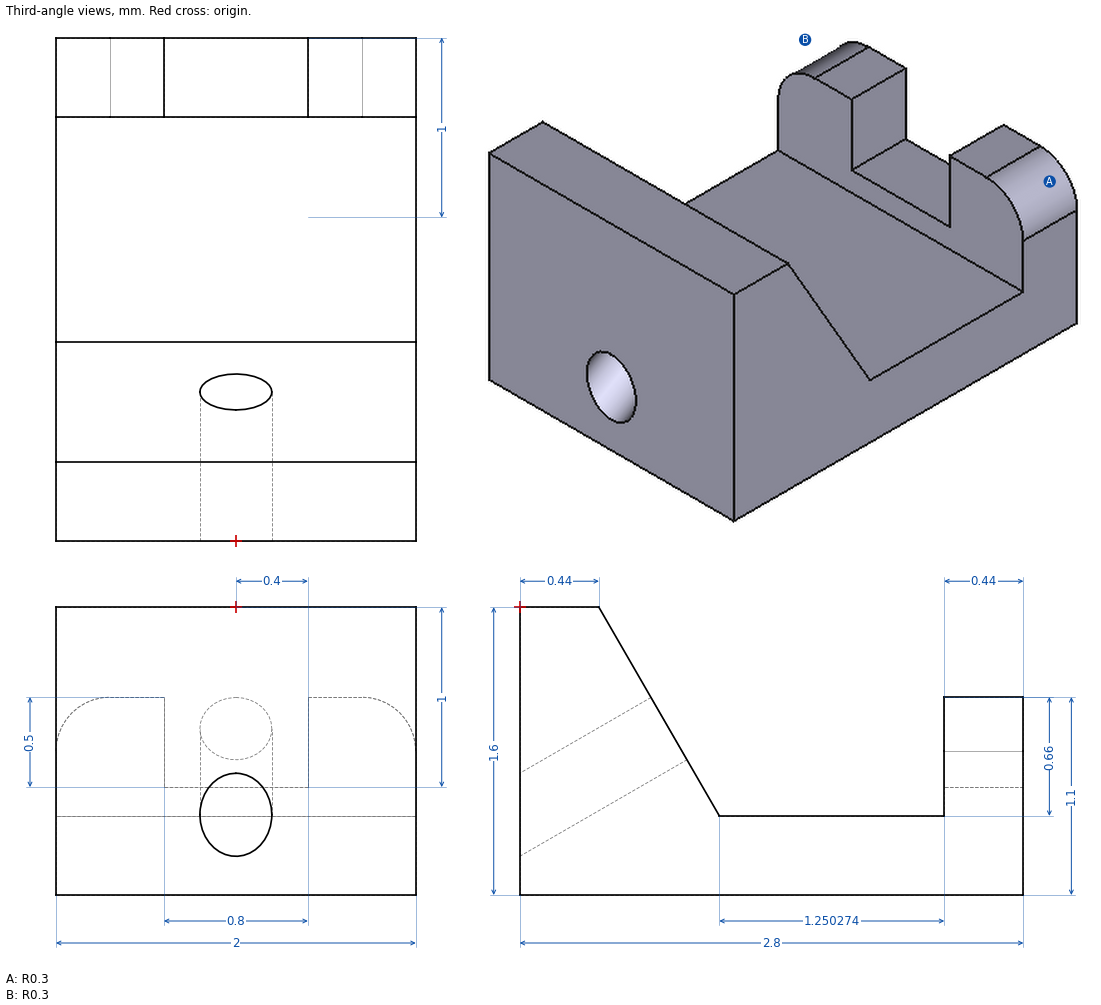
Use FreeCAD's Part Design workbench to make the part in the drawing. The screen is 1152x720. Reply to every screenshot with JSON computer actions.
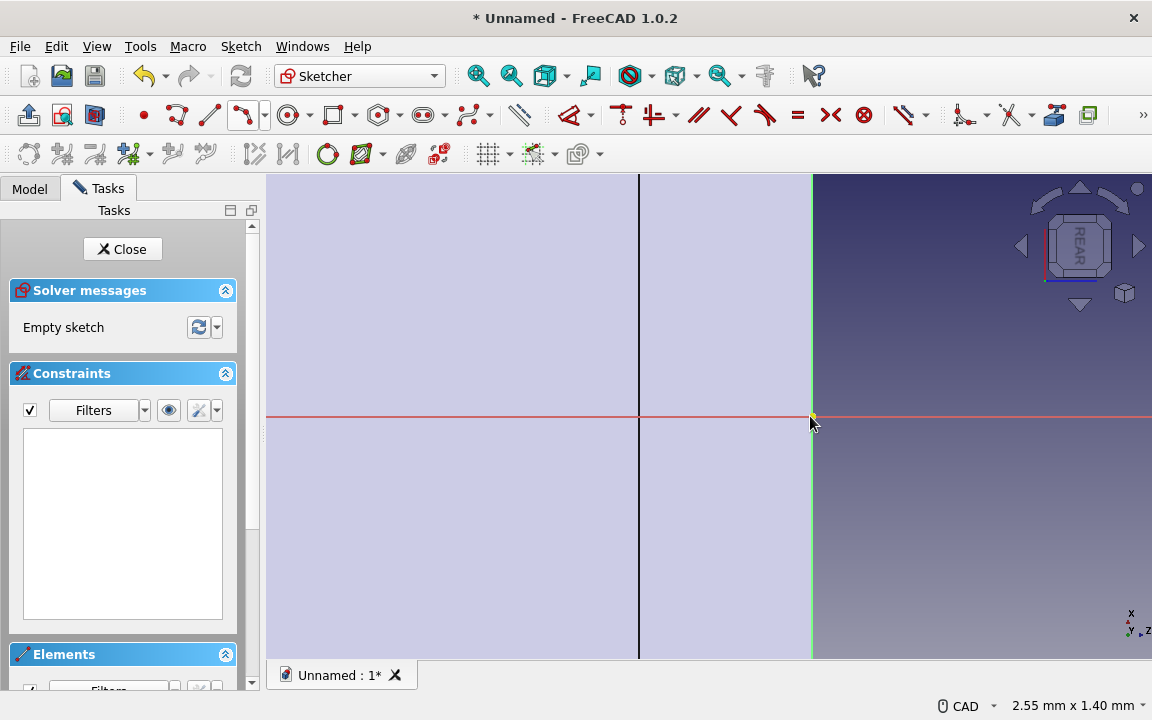
{"action": "left_click", "coordinate": [332, 116]}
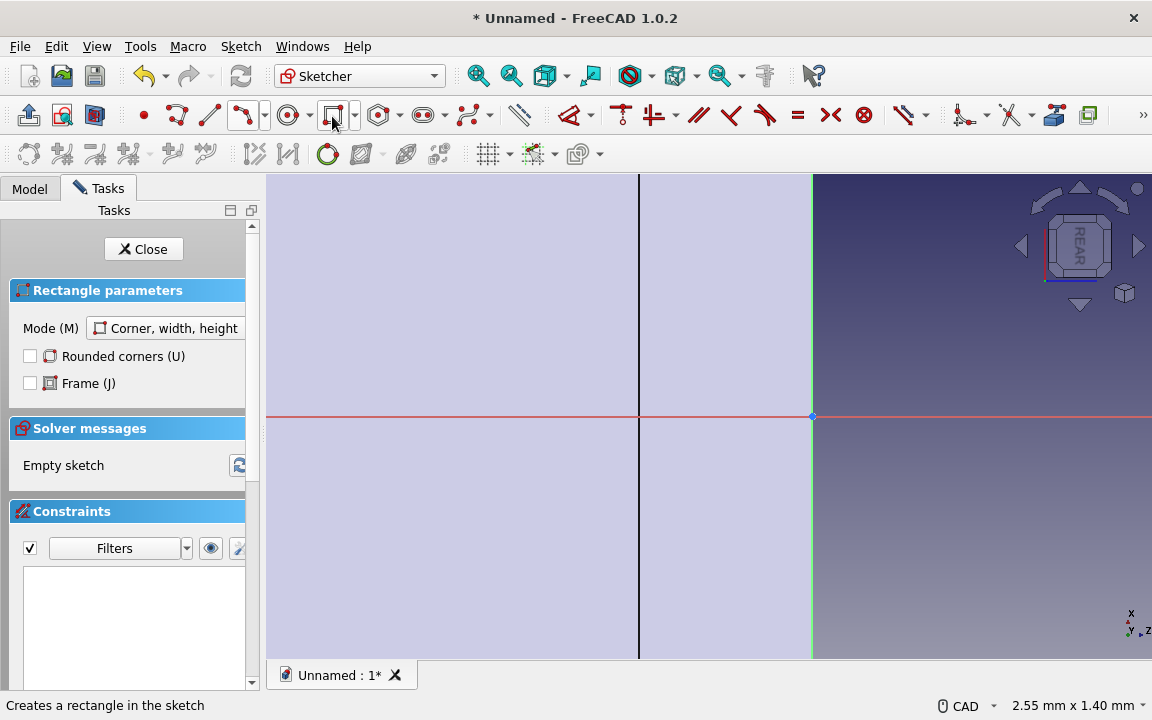
{"action": "left_click", "coordinate": [465, 278]}
{"action": "left_click", "coordinate": [639, 555]}
{"action": "key", "text": "Escape"}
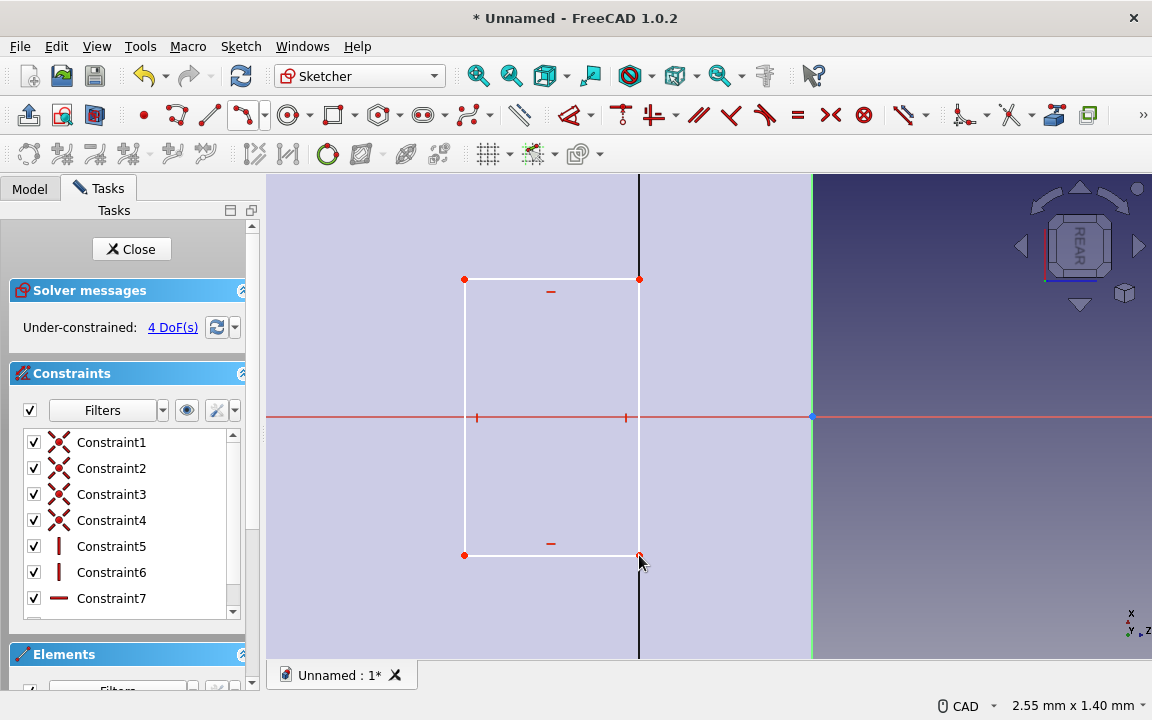
{"action": "left_click", "coordinate": [568, 116]}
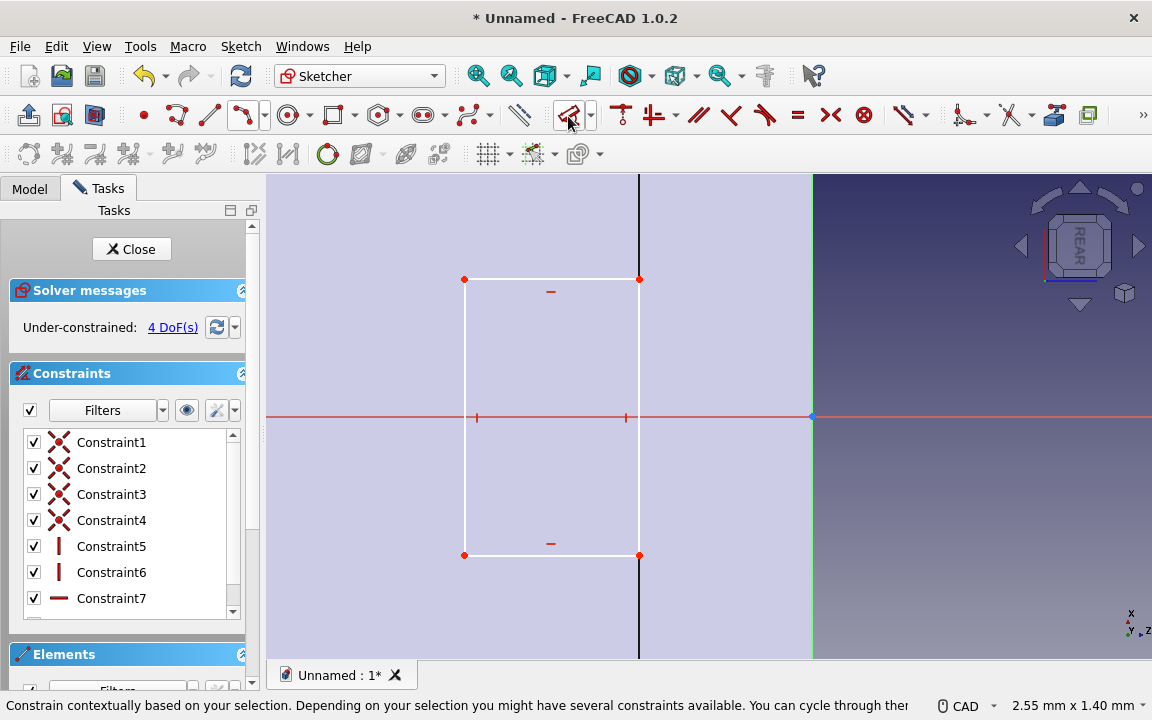
{"action": "left_click", "coordinate": [465, 279]}
{"action": "left_click", "coordinate": [639, 245]}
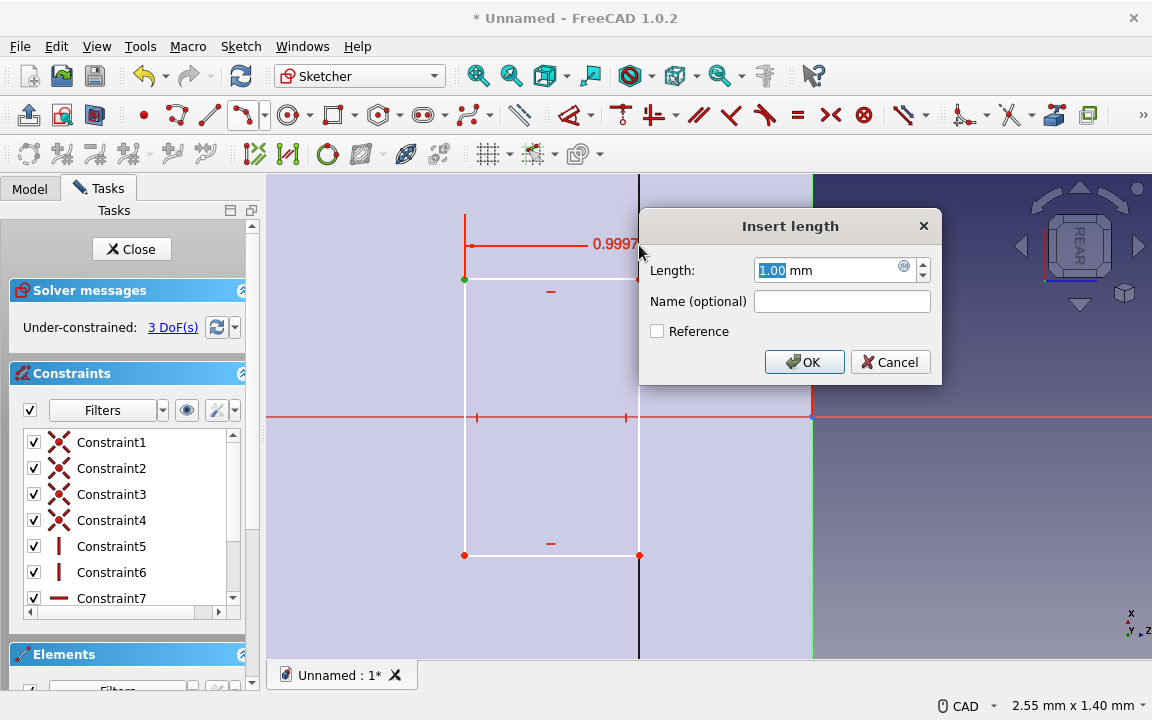
{"action": "type", "text": "1"}
{"action": "key", "text": "Return"}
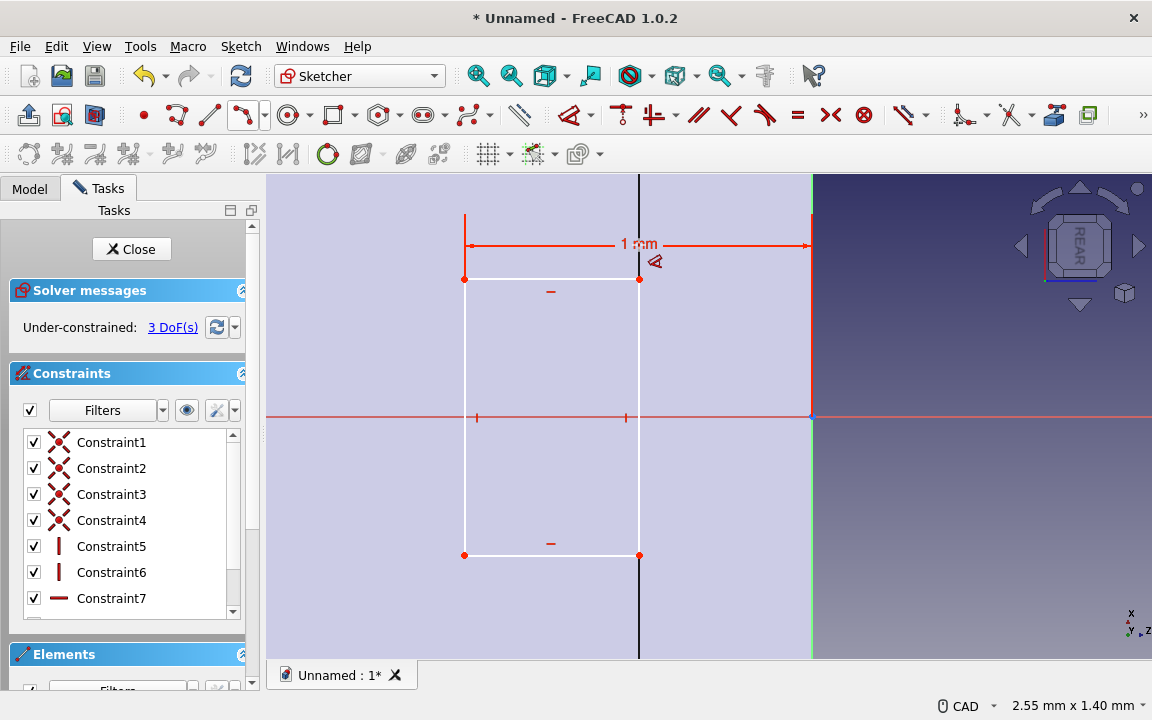
{"action": "left_click", "coordinate": [465, 362]}
{"action": "left_click", "coordinate": [431, 354]}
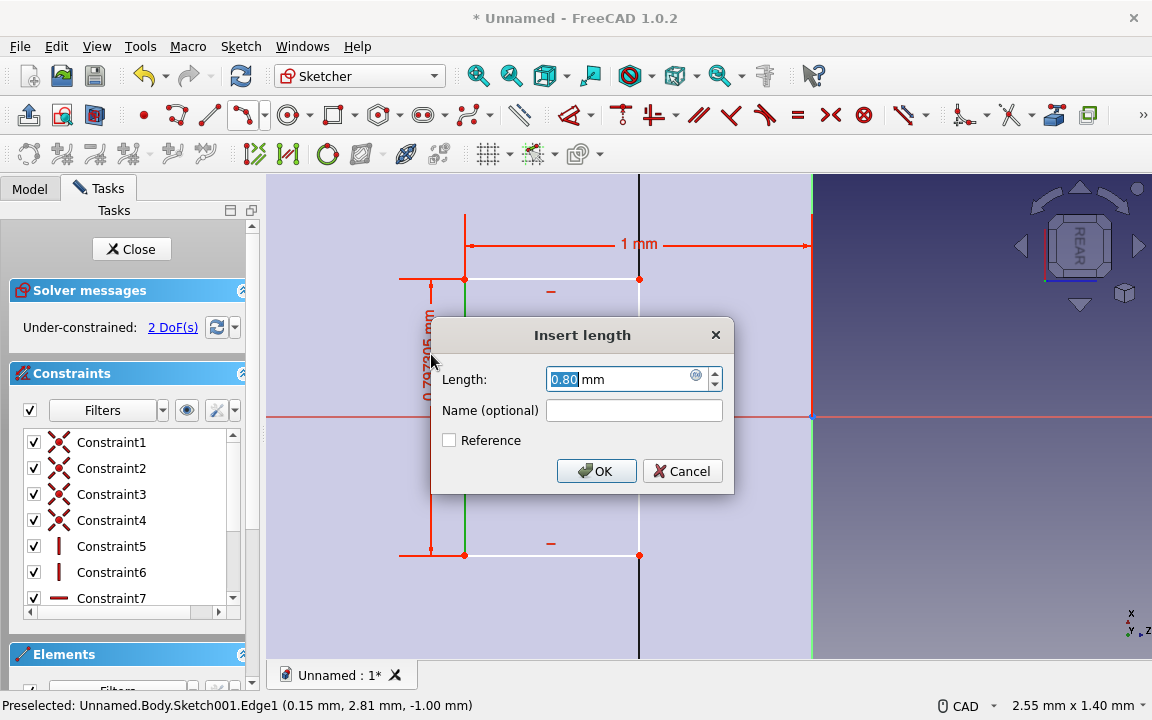
{"action": "type", "text": "0.8"}
{"action": "key", "text": "Return"}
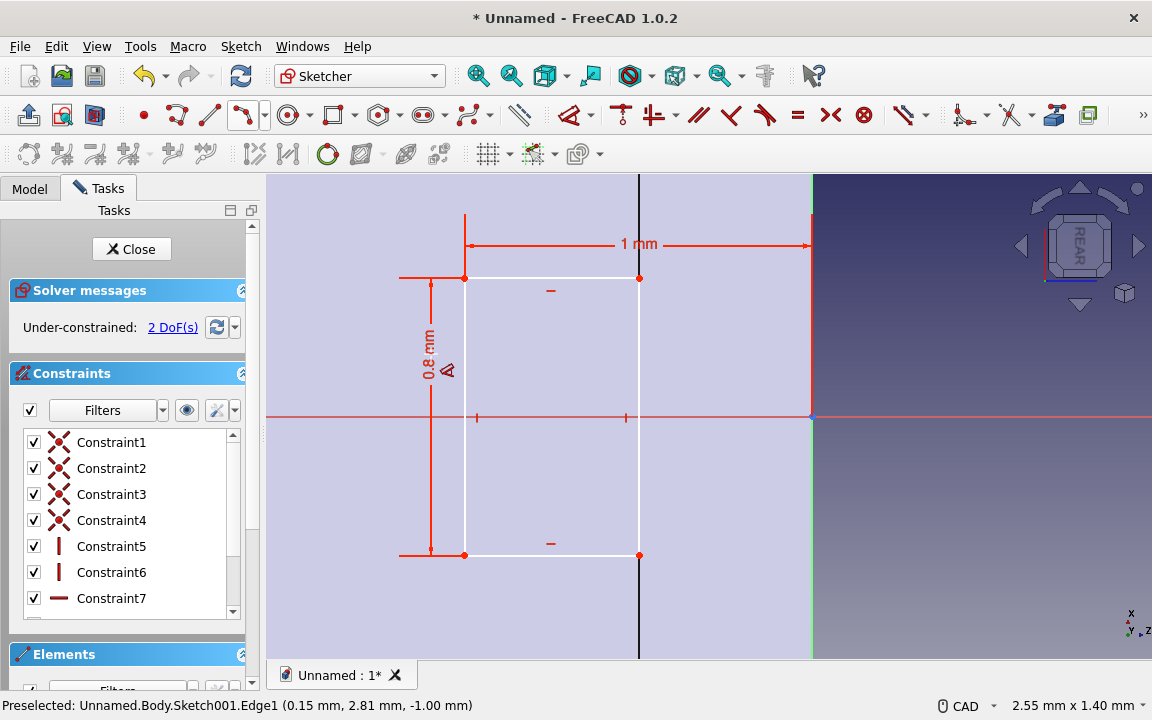
{"action": "left_click", "coordinate": [517, 556]}
{"action": "left_click", "coordinate": [552, 590]}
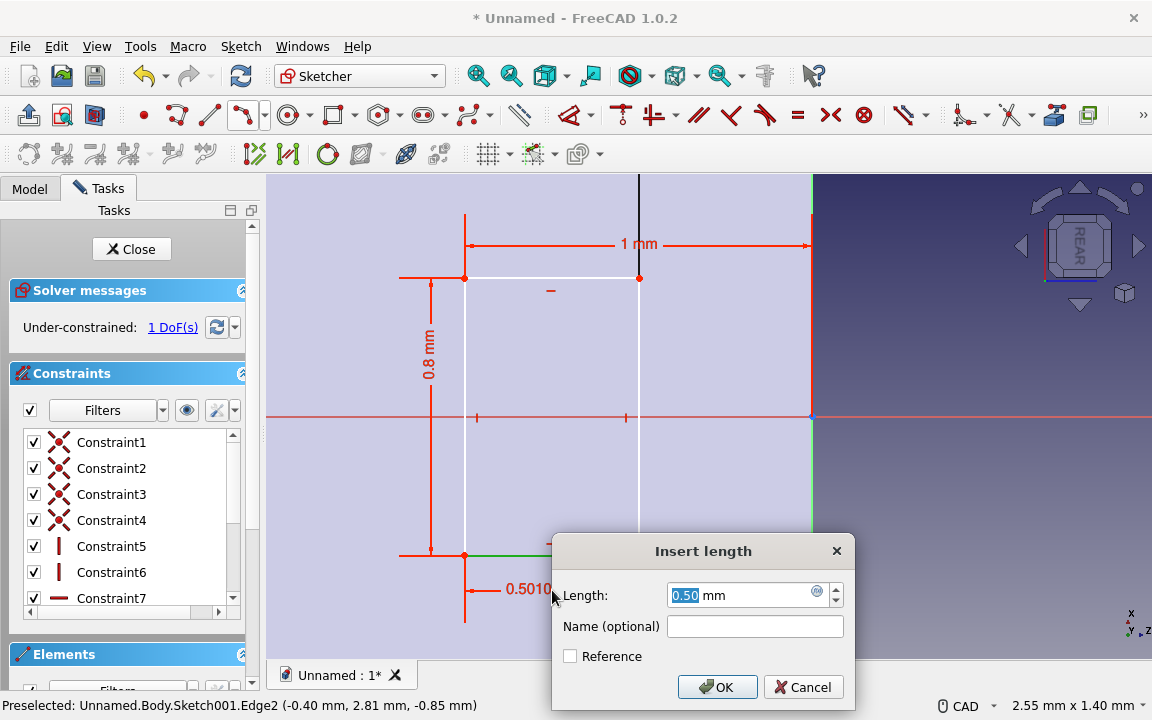
{"action": "type", "text": "0.5"}
{"action": "key", "text": "Return"}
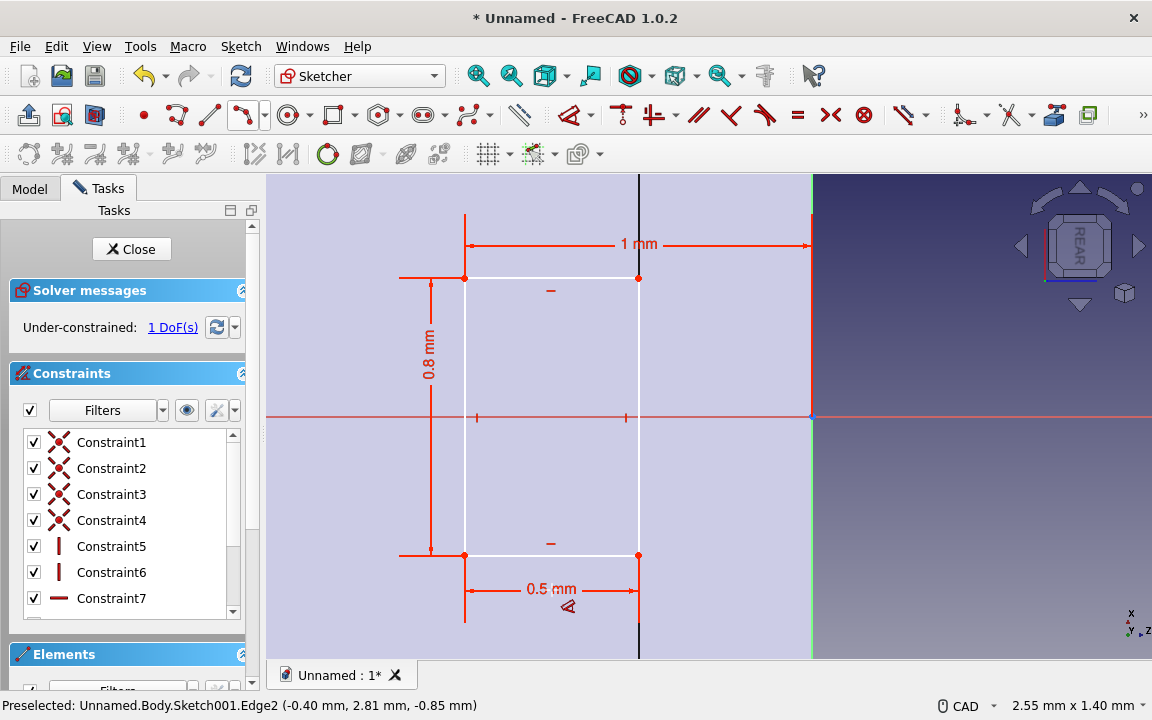
{"action": "left_click", "coordinate": [465, 278]}
{"action": "left_click", "coordinate": [846, 347]}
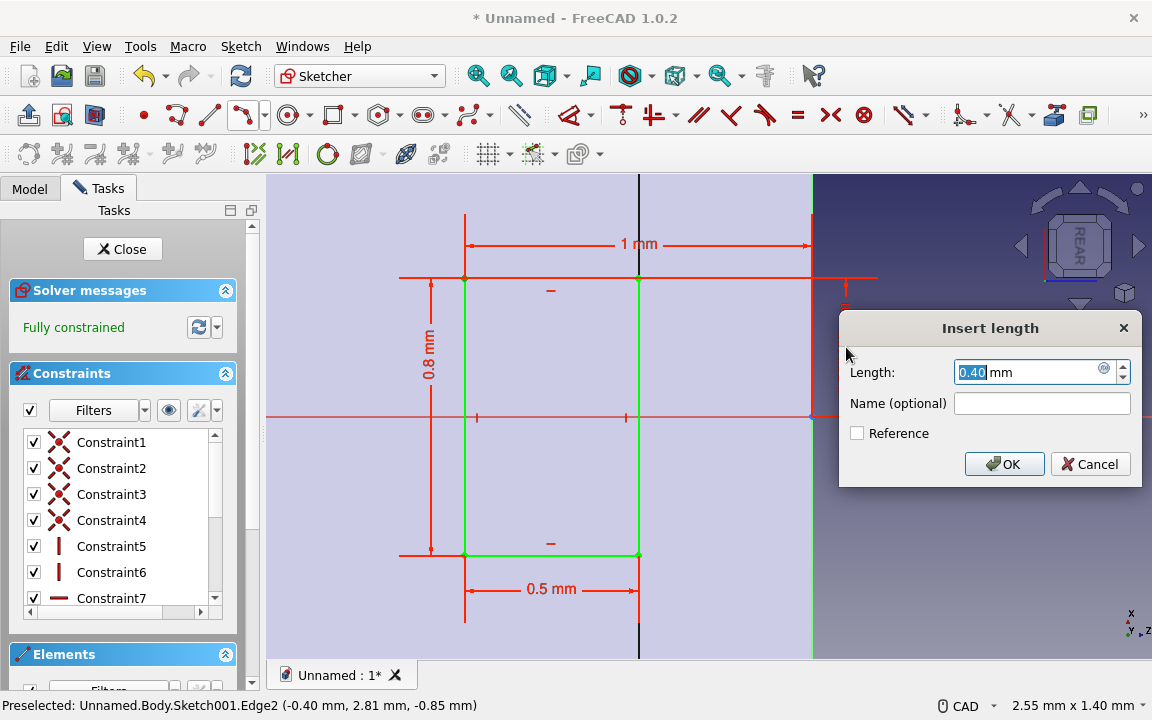
{"action": "type", "text": "0.4"}
{"action": "key", "text": "Return"}
{"action": "key", "text": "Escape"}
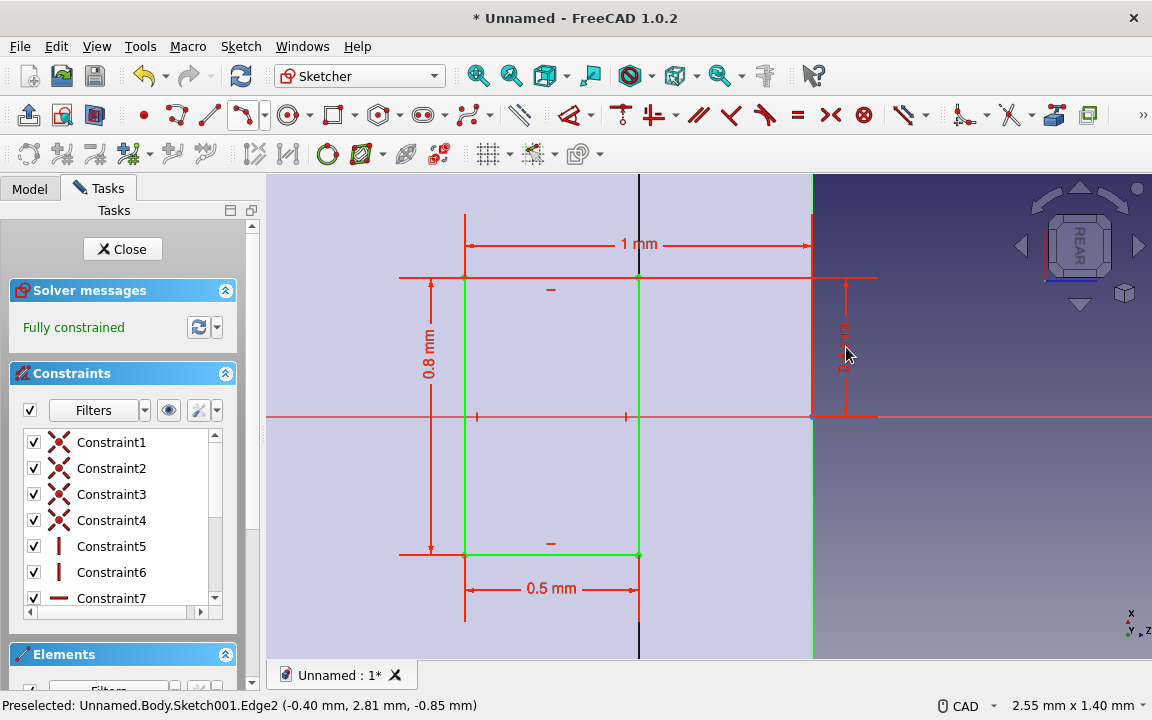
{"action": "left_click", "coordinate": [123, 249]}